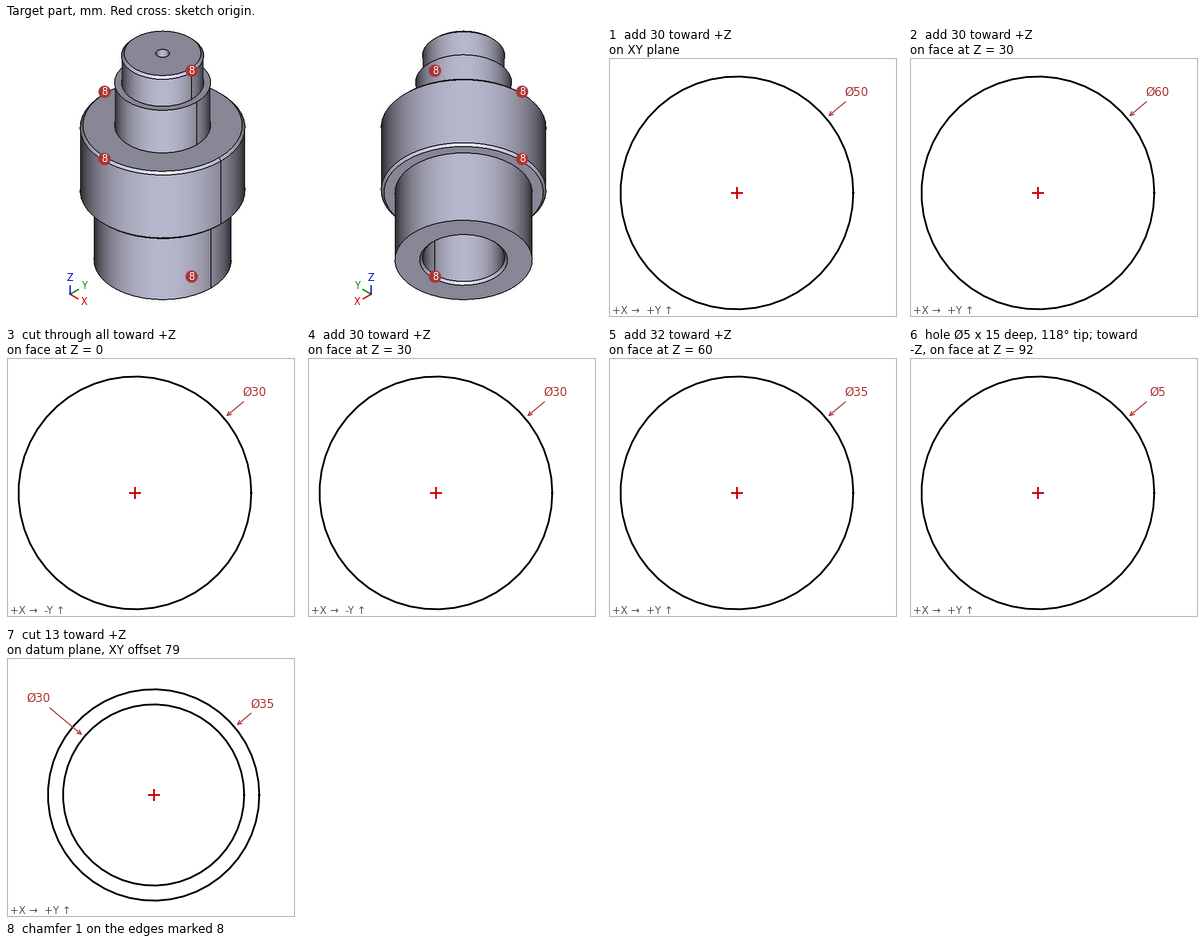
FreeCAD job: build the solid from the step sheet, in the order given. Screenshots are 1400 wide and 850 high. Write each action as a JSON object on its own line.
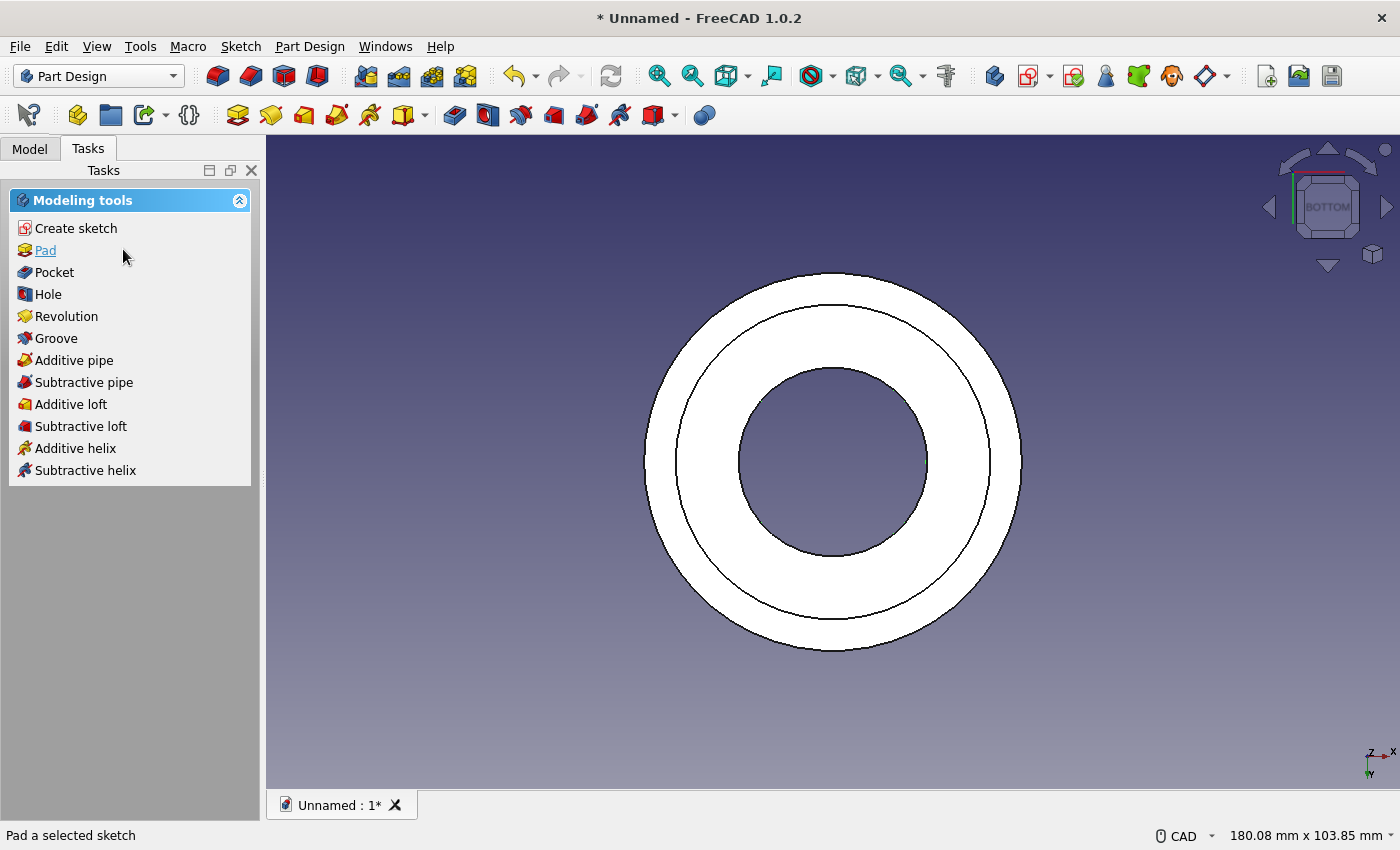
{"action": "left_click", "coordinate": [238, 116]}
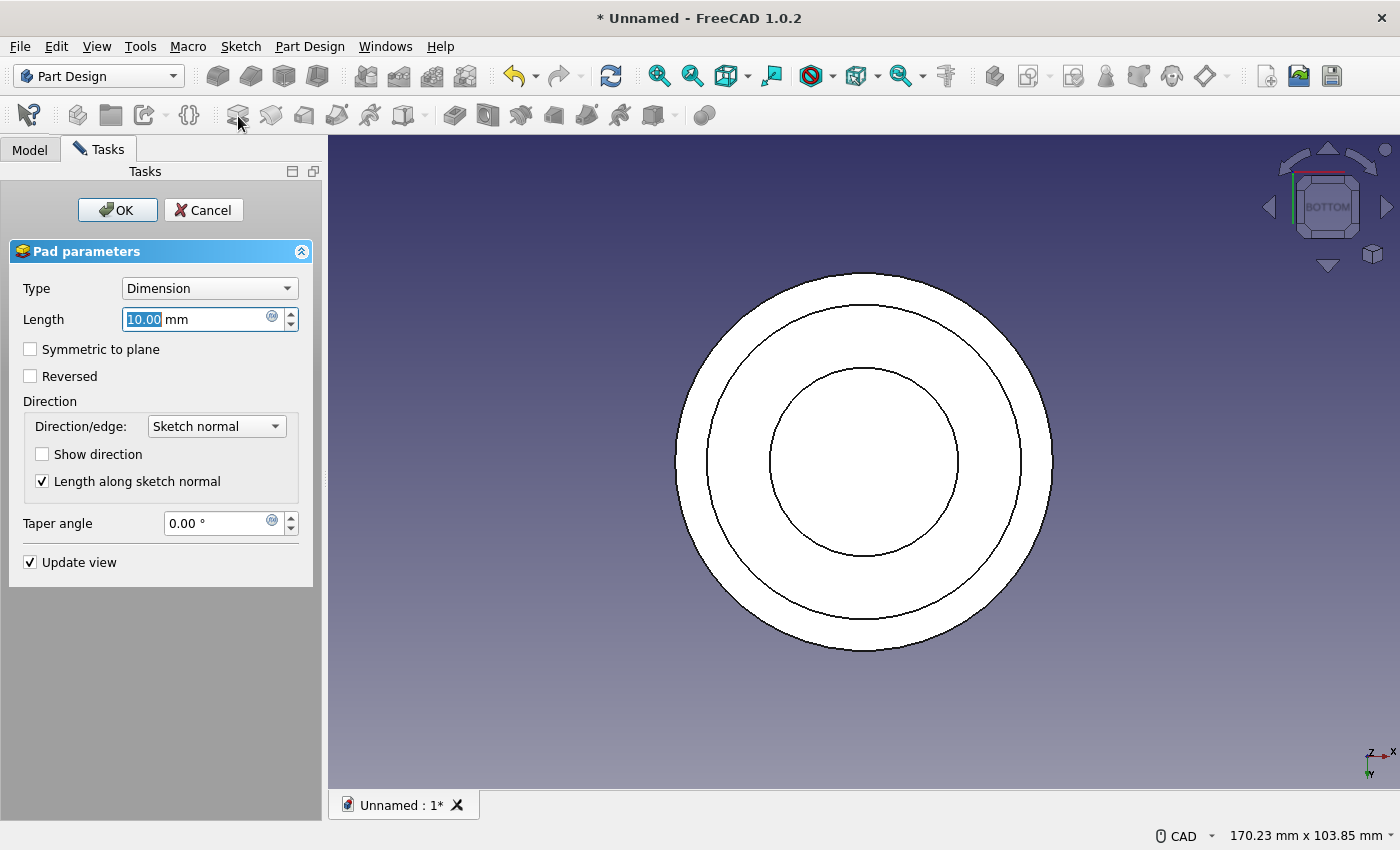
{"action": "type", "text": "30"}
{"action": "key", "text": "Tab"}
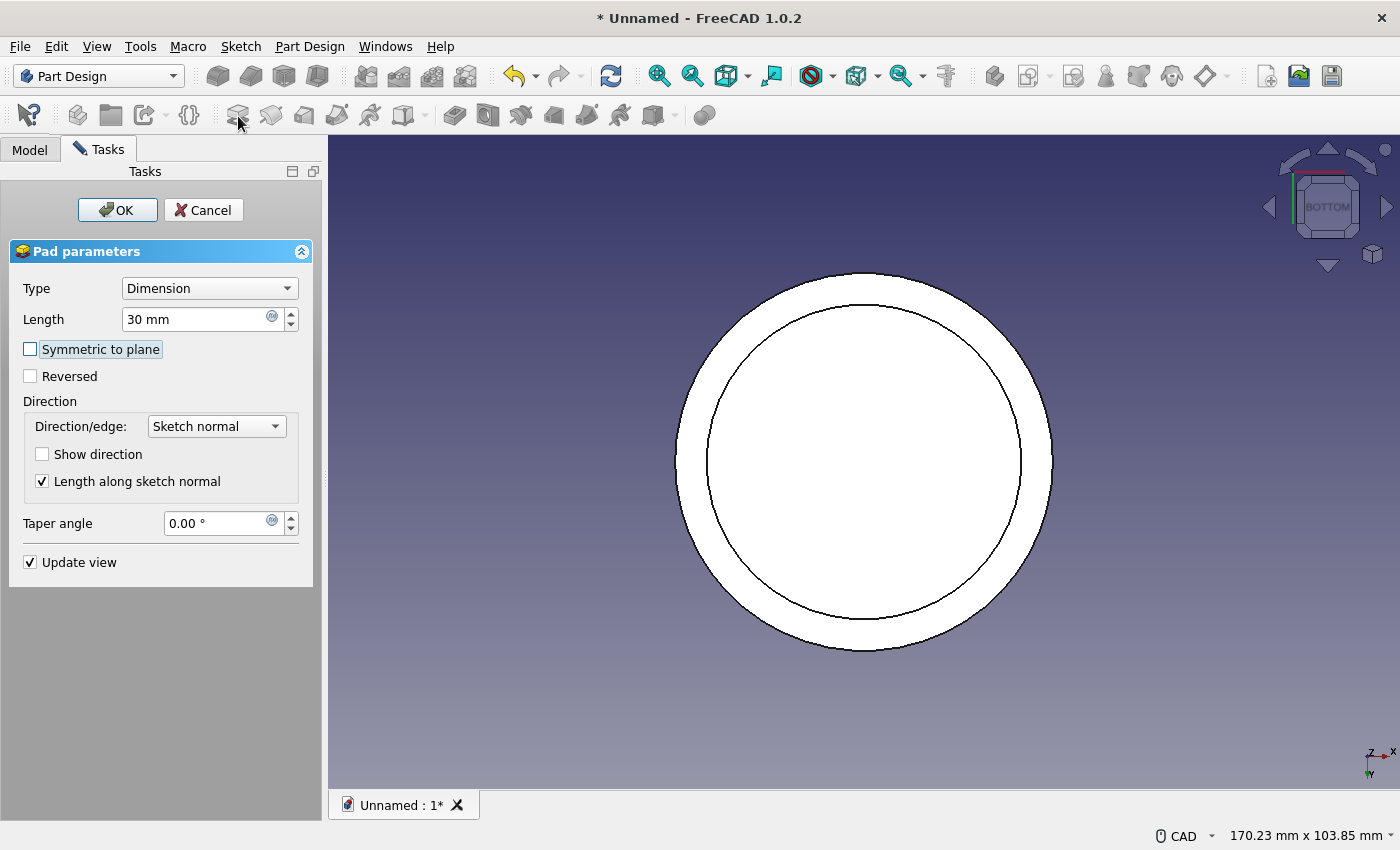
{"action": "left_click", "coordinate": [31, 376]}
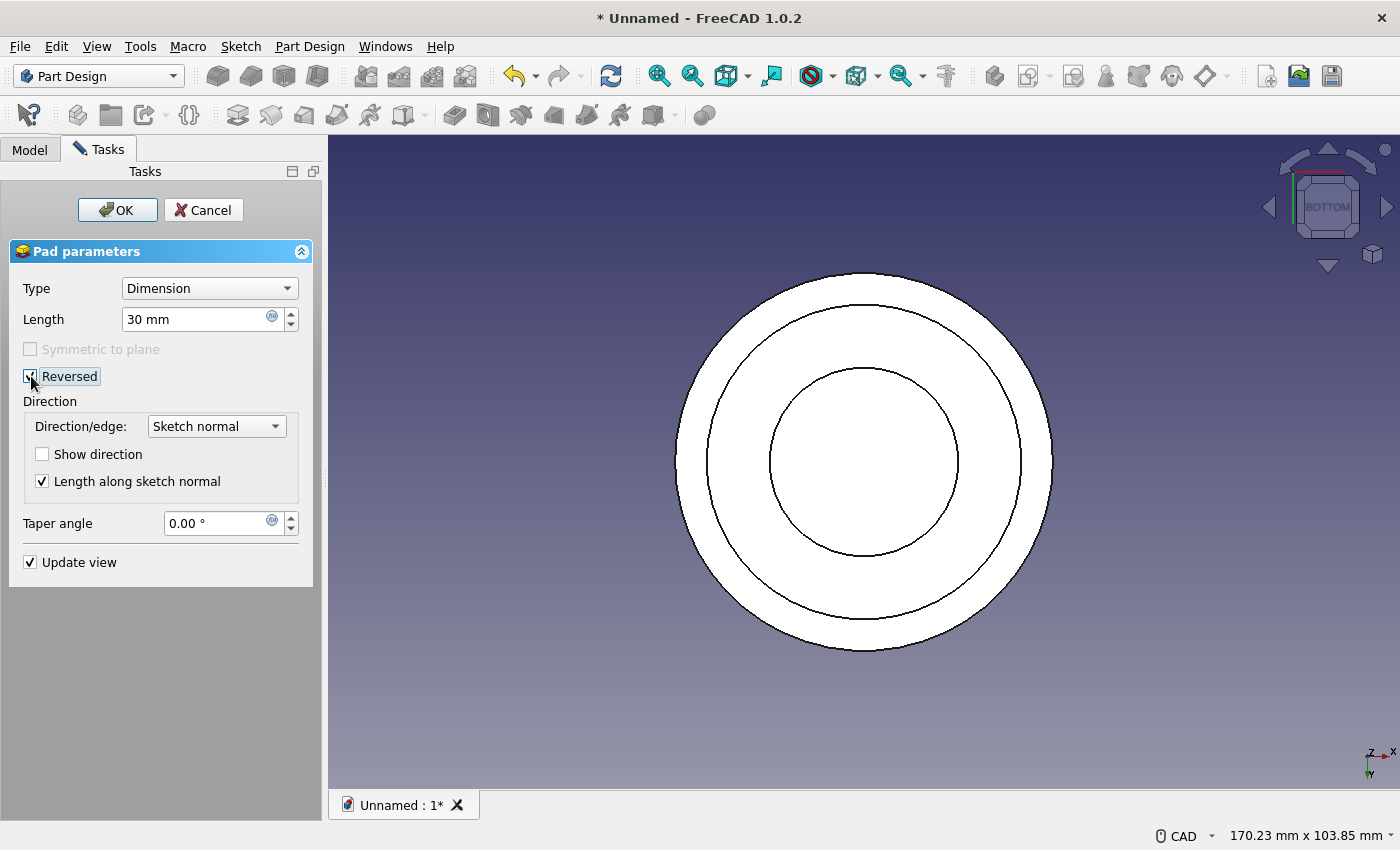
{"action": "left_click", "coordinate": [118, 210]}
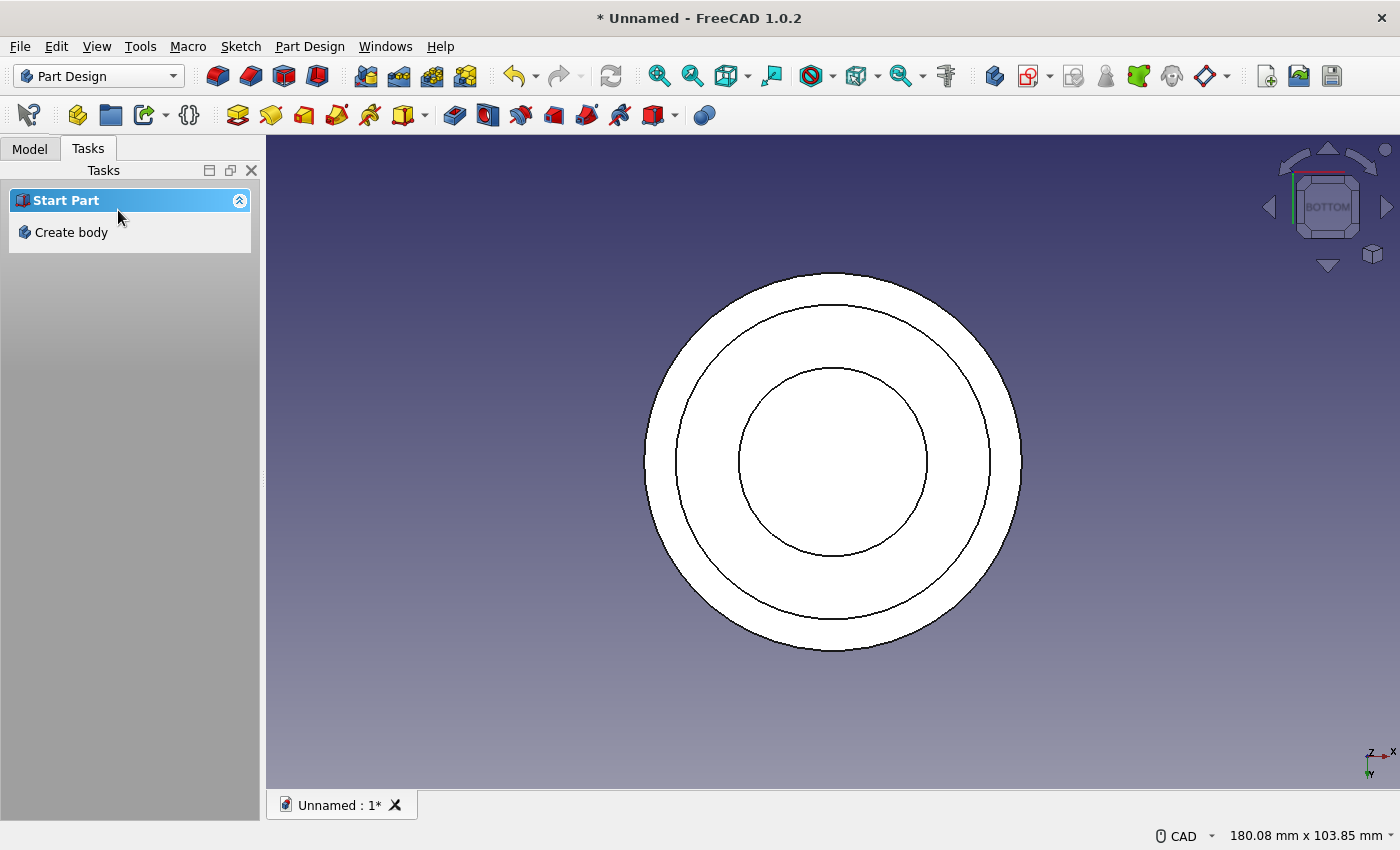
{"action": "key", "text": "0"}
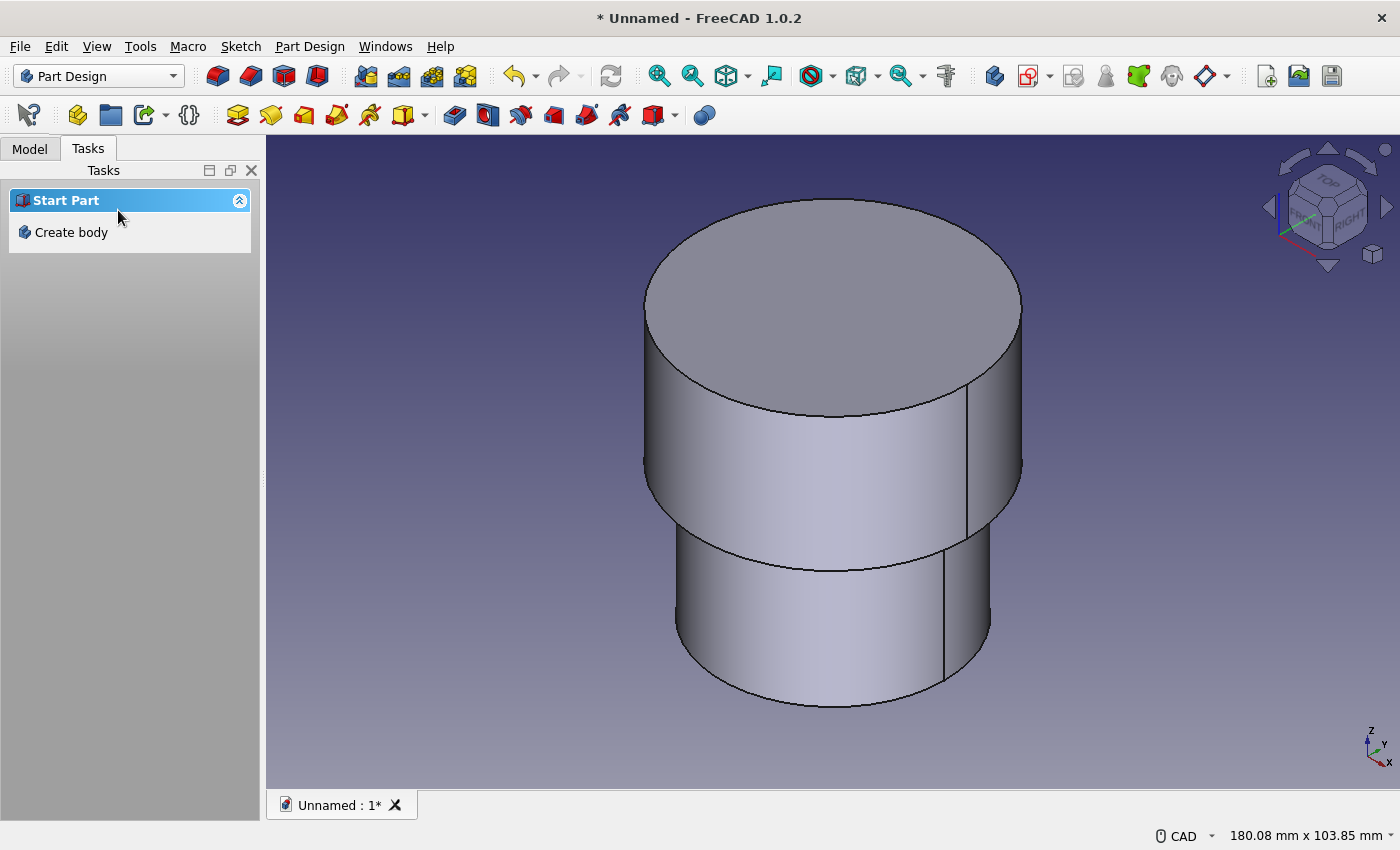
{"action": "left_click", "coordinate": [833, 307]}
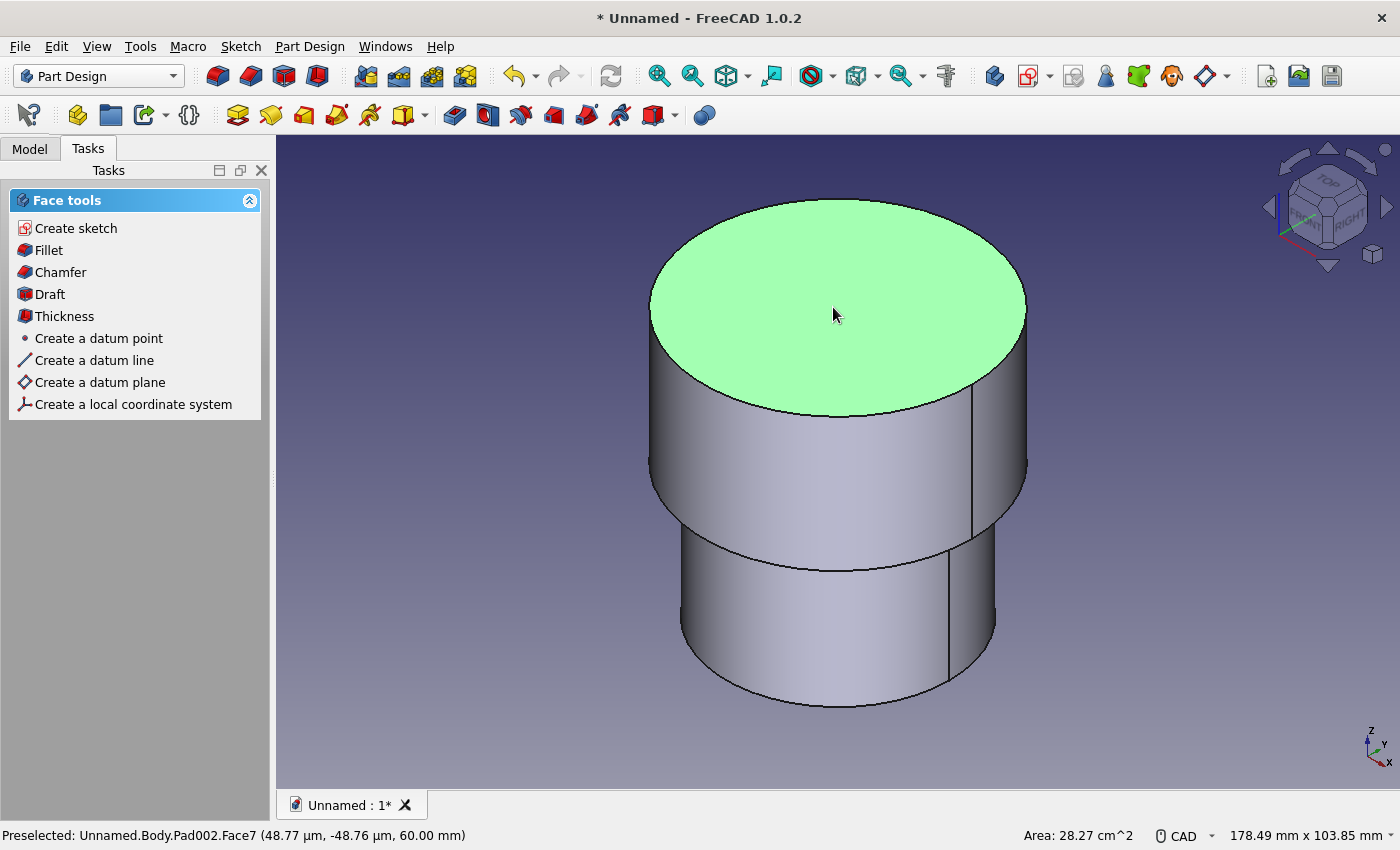
{"action": "left_click", "coordinate": [1028, 76]}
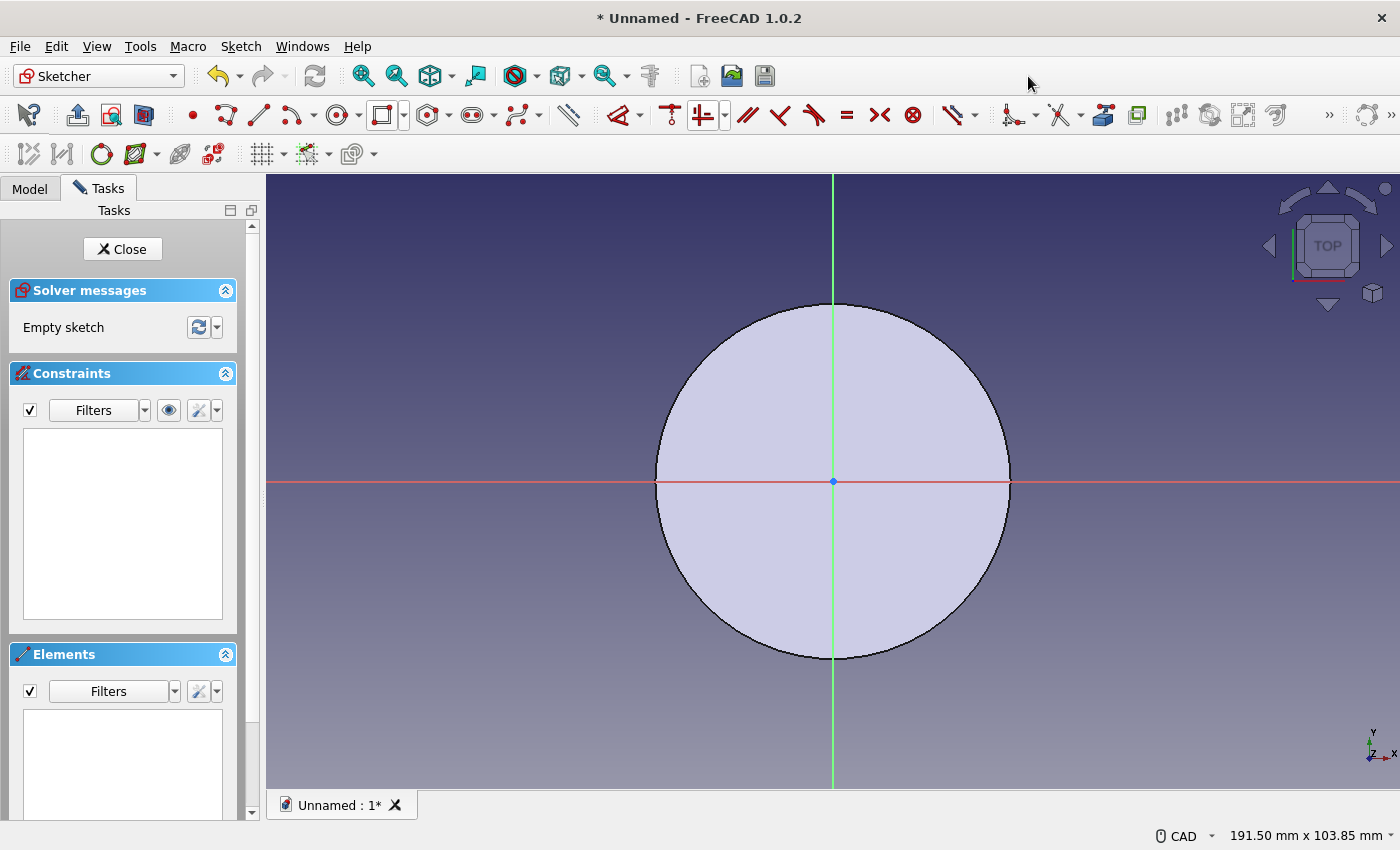
{"action": "scroll", "coordinate": [916, 481], "scroll_direction": "up", "scroll_amount": 3}